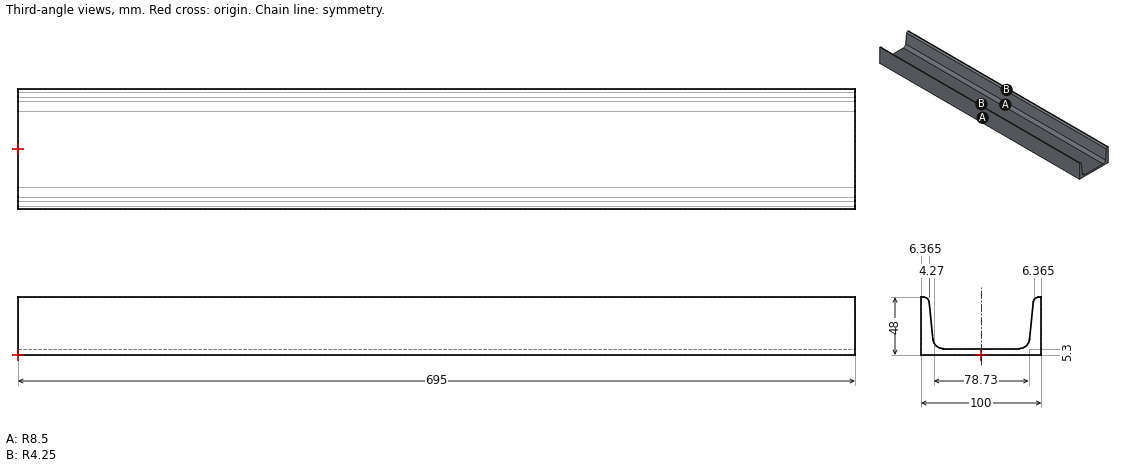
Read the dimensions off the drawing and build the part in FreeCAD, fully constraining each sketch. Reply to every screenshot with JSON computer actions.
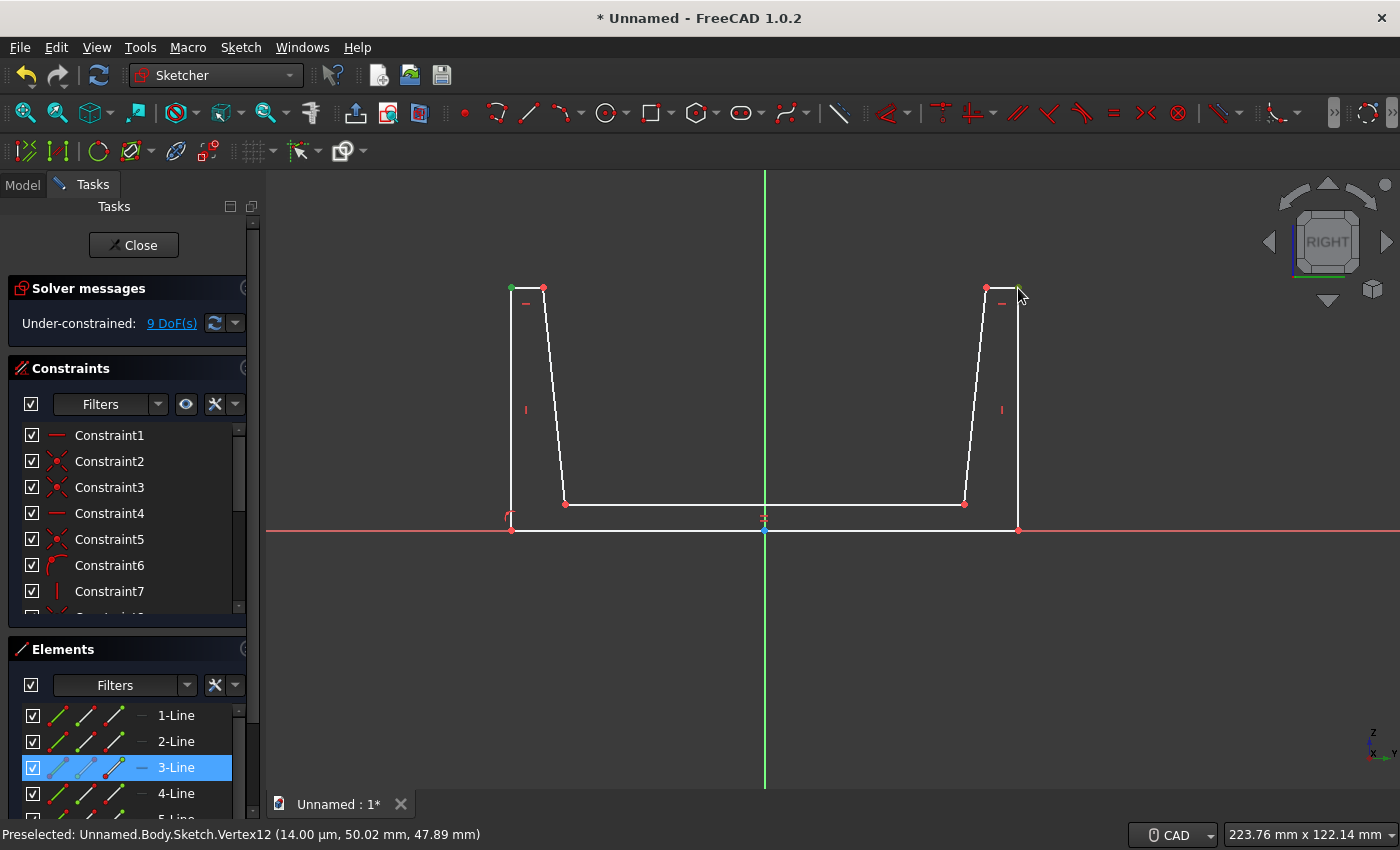
{"action": "left_click", "coordinate": [765, 721]}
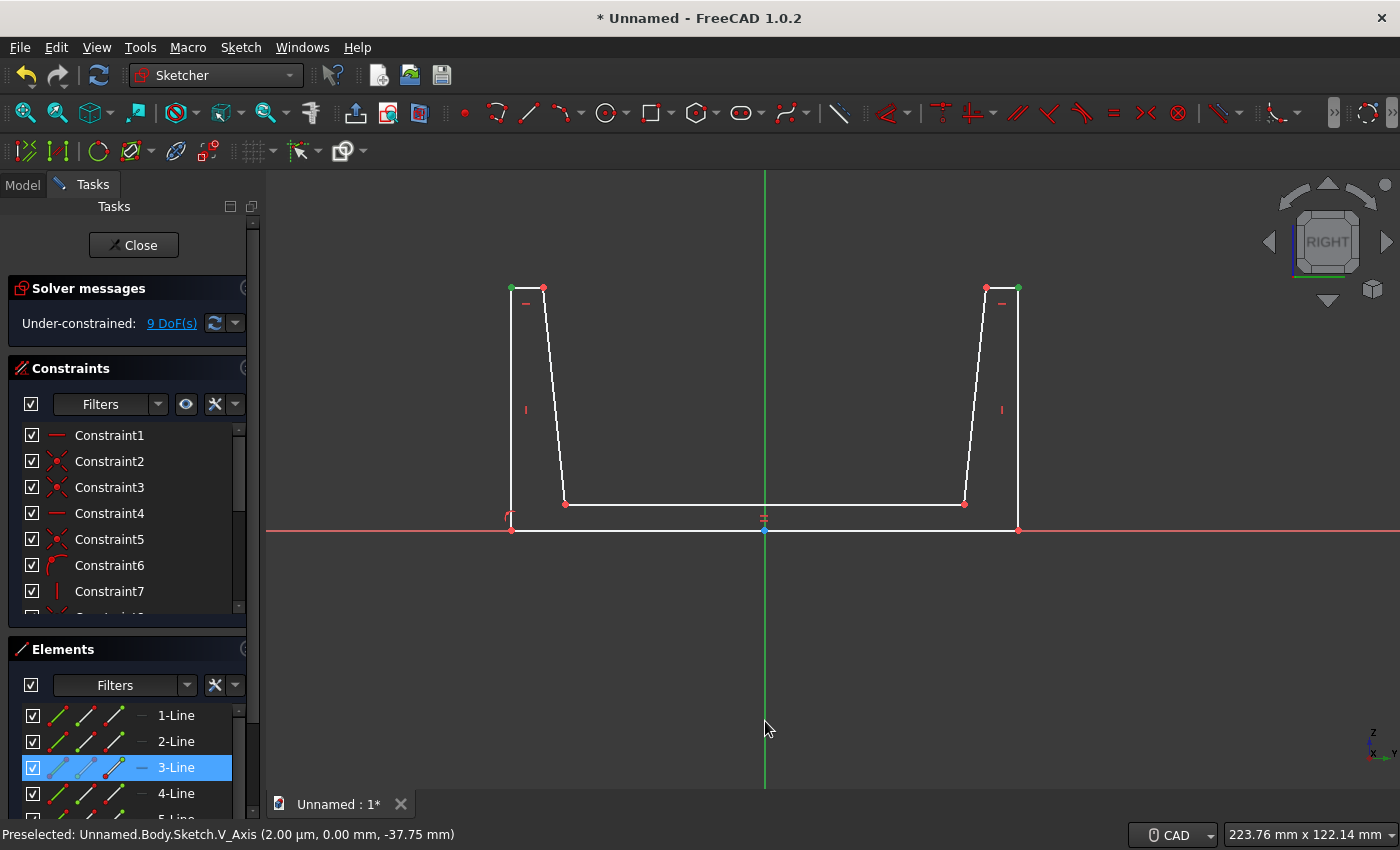
{"action": "key", "text": "s"}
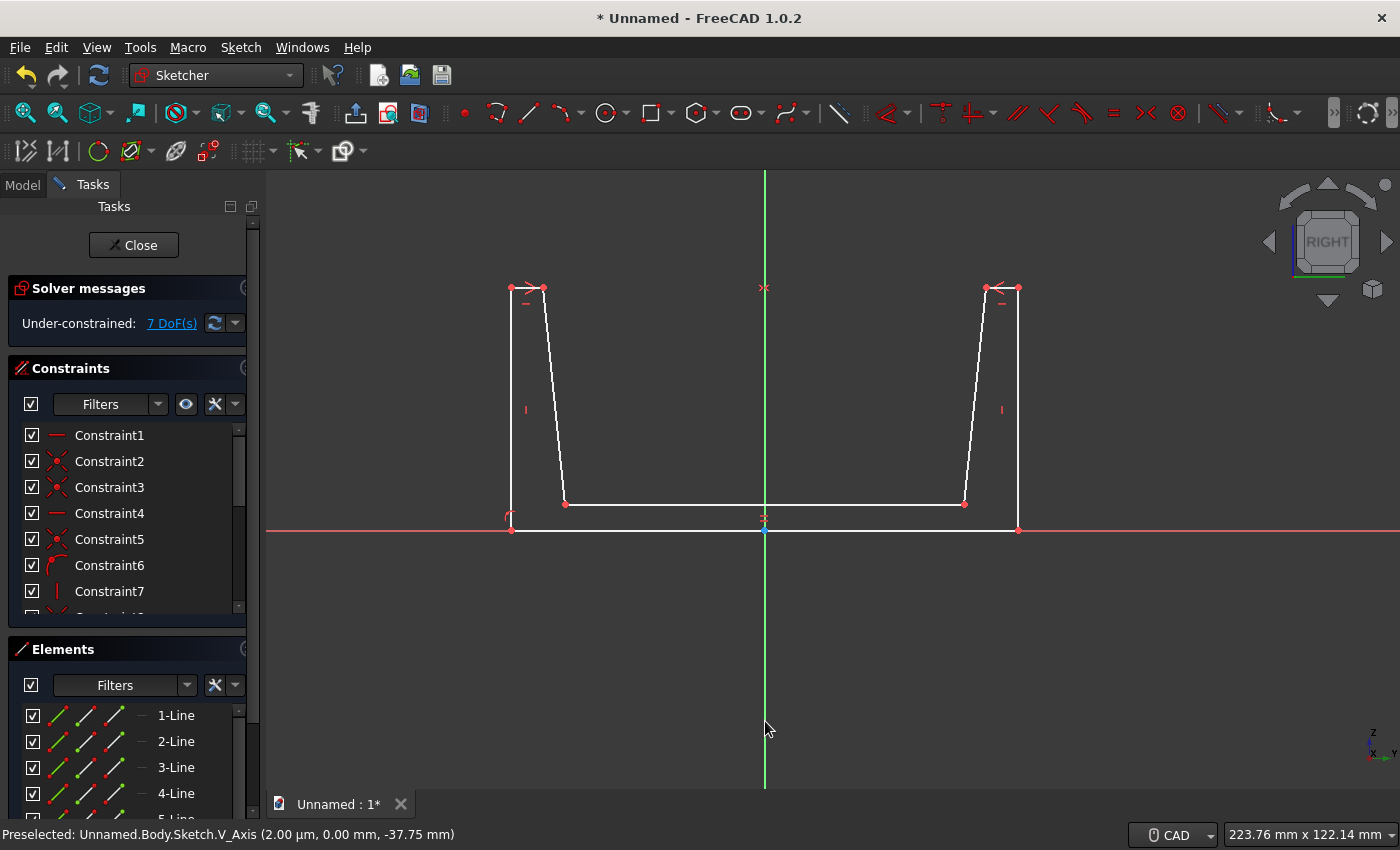
{"action": "left_click", "coordinate": [886, 114]}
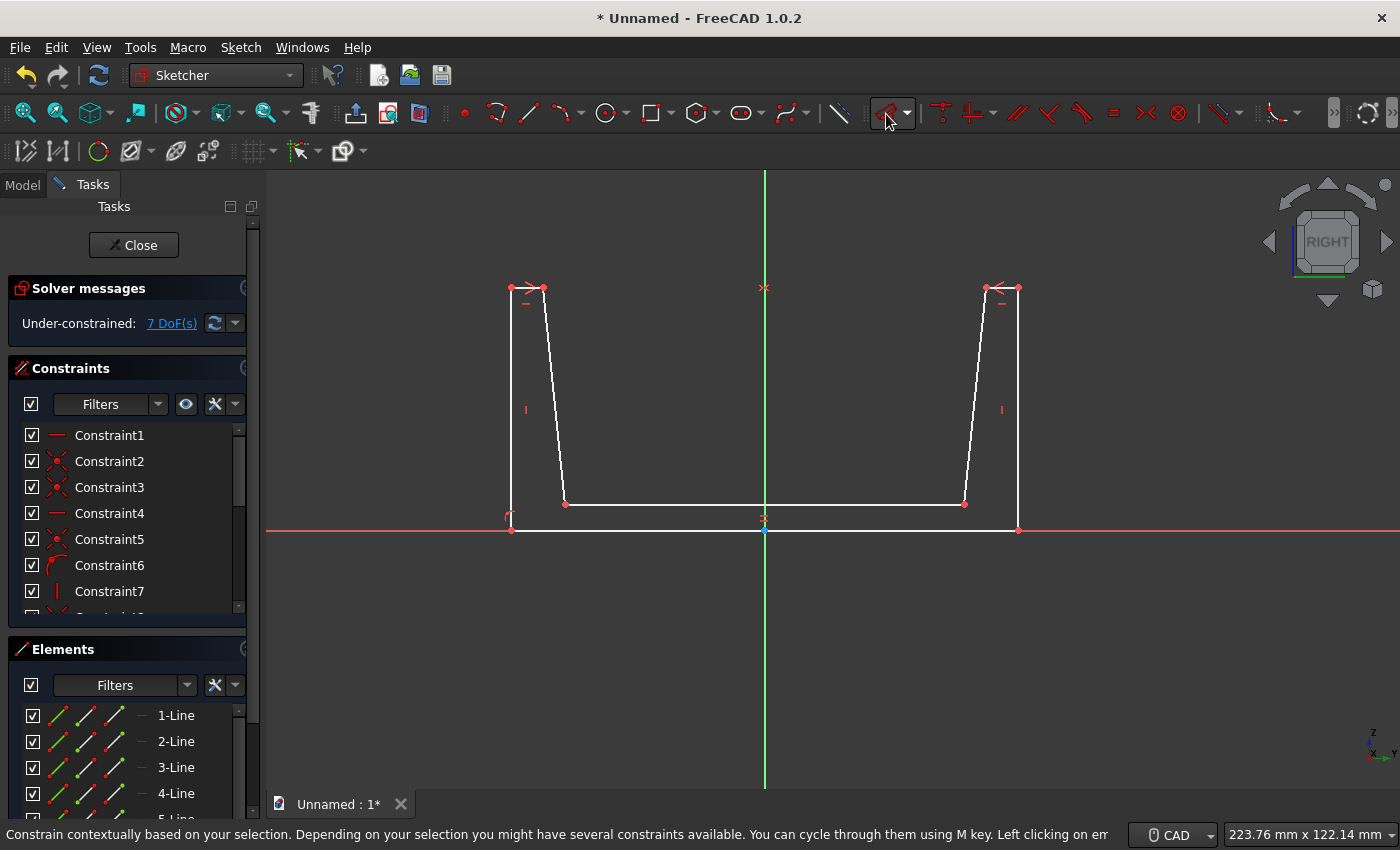
{"action": "left_click", "coordinate": [511, 361]}
{"action": "left_click", "coordinate": [477, 409]}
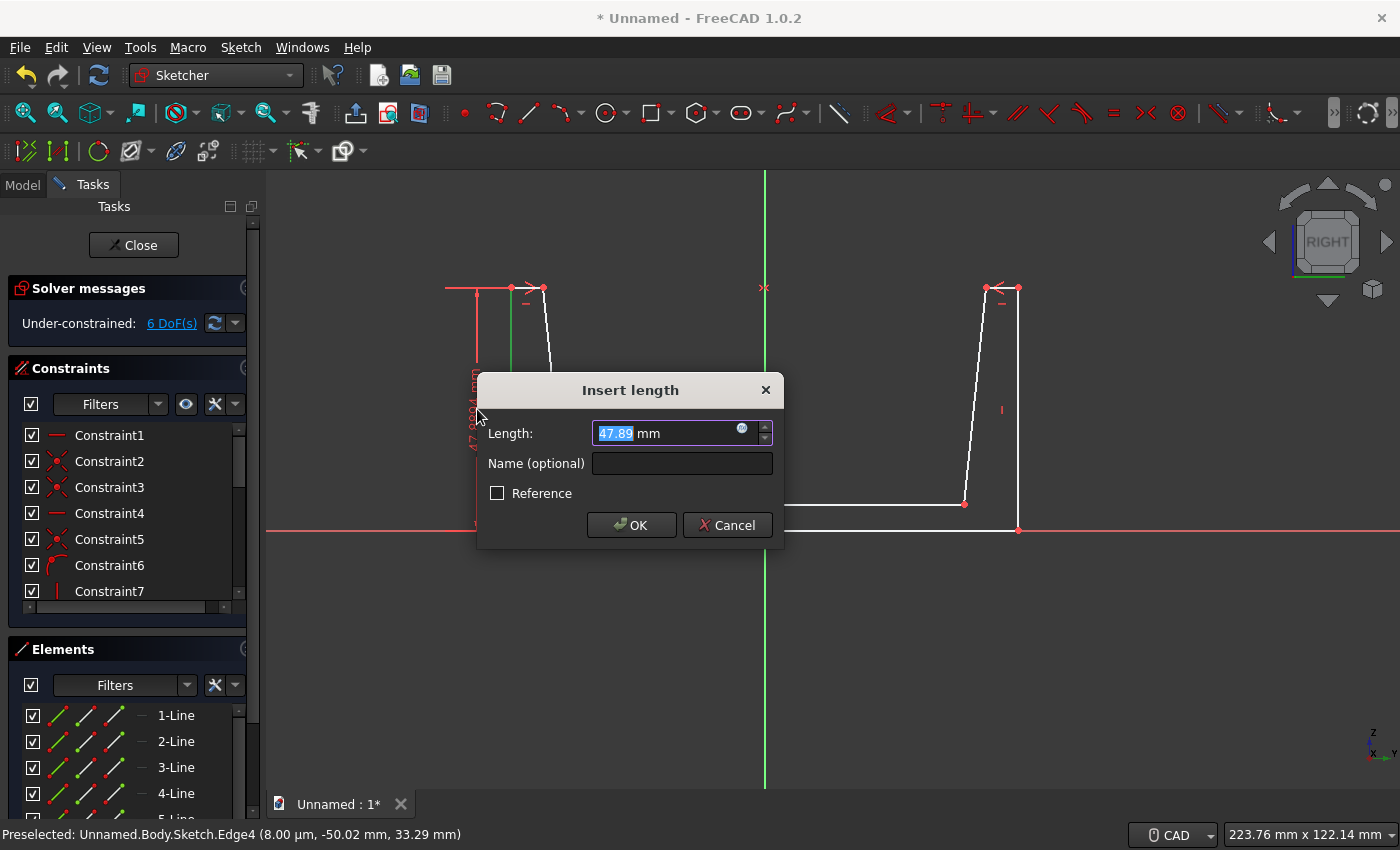
{"action": "type", "text": "48"}
{"action": "key", "text": "Return"}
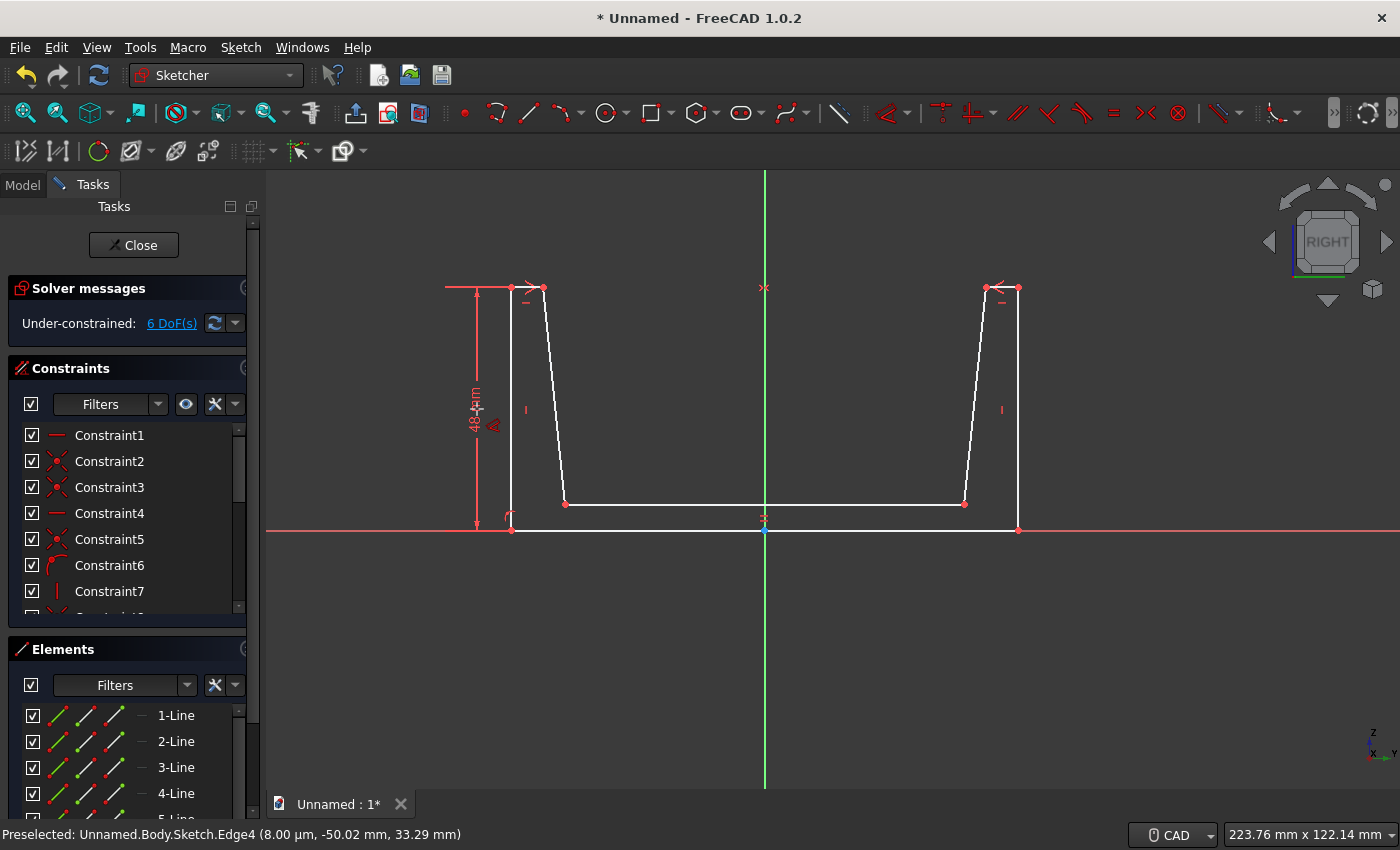
{"action": "left_click", "coordinate": [663, 531]}
{"action": "left_click", "coordinate": [648, 565]}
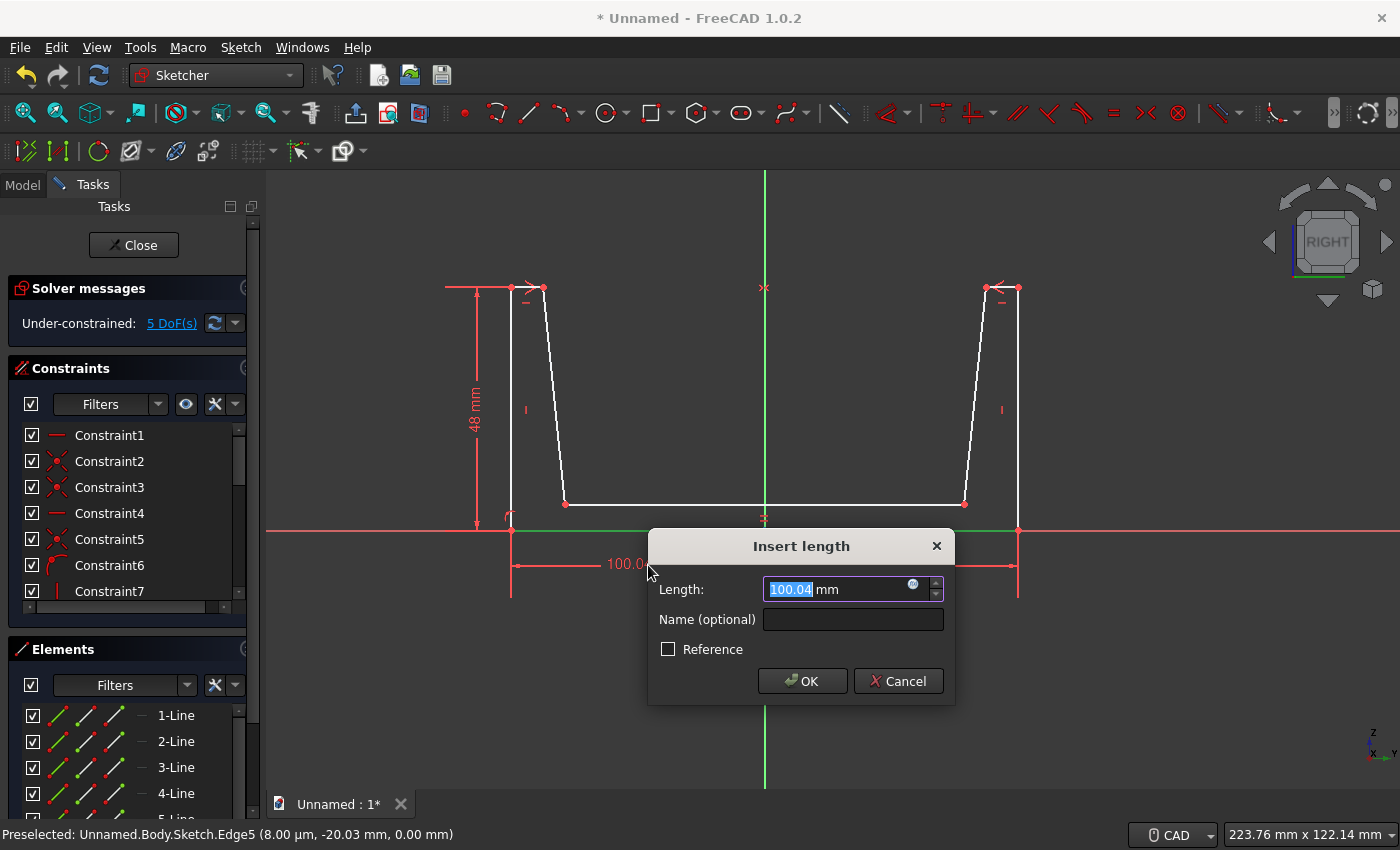
{"action": "type", "text": "100"}
{"action": "key", "text": "Return"}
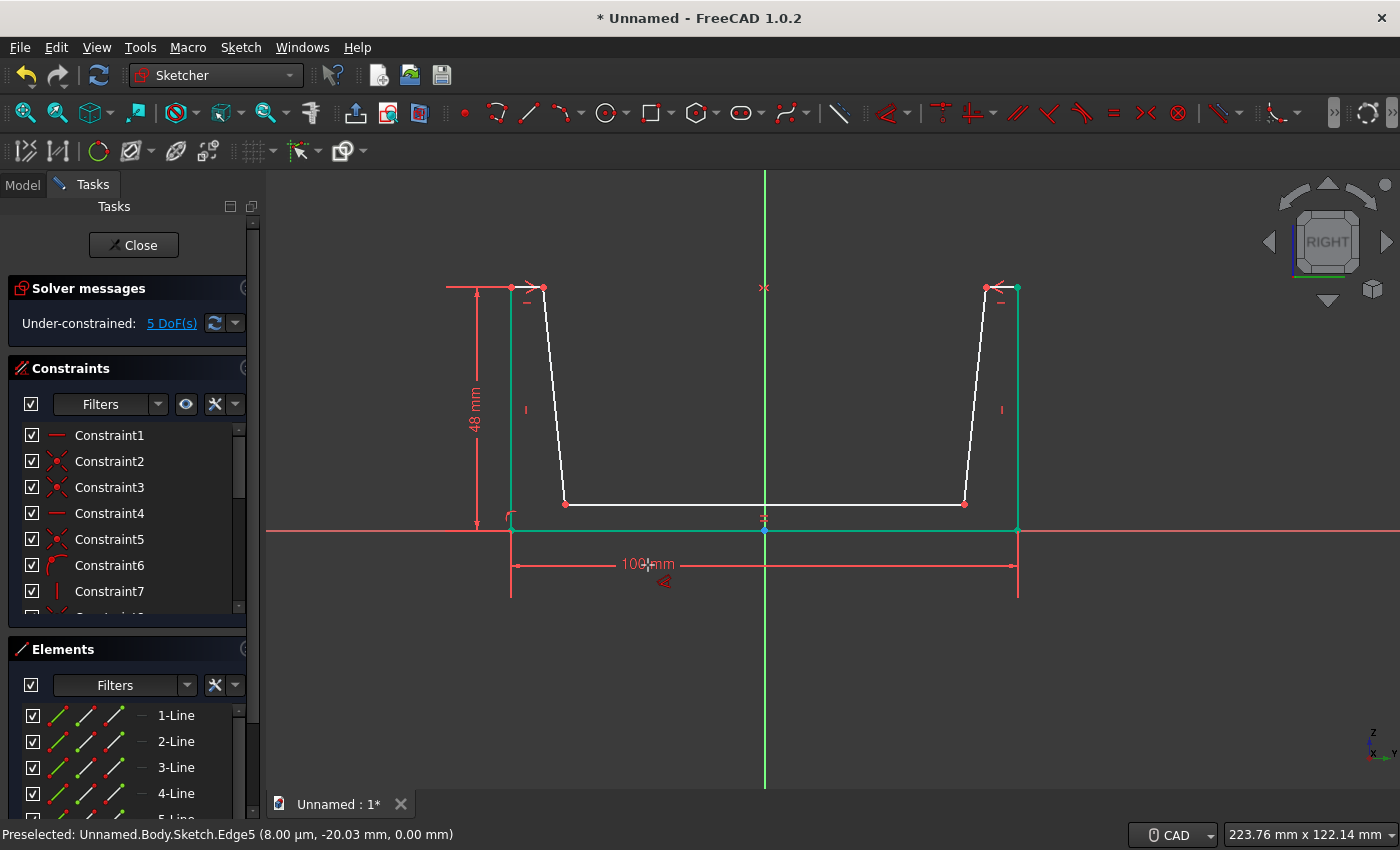
{"action": "scroll", "coordinate": [964, 505], "scroll_direction": "up", "scroll_amount": 2}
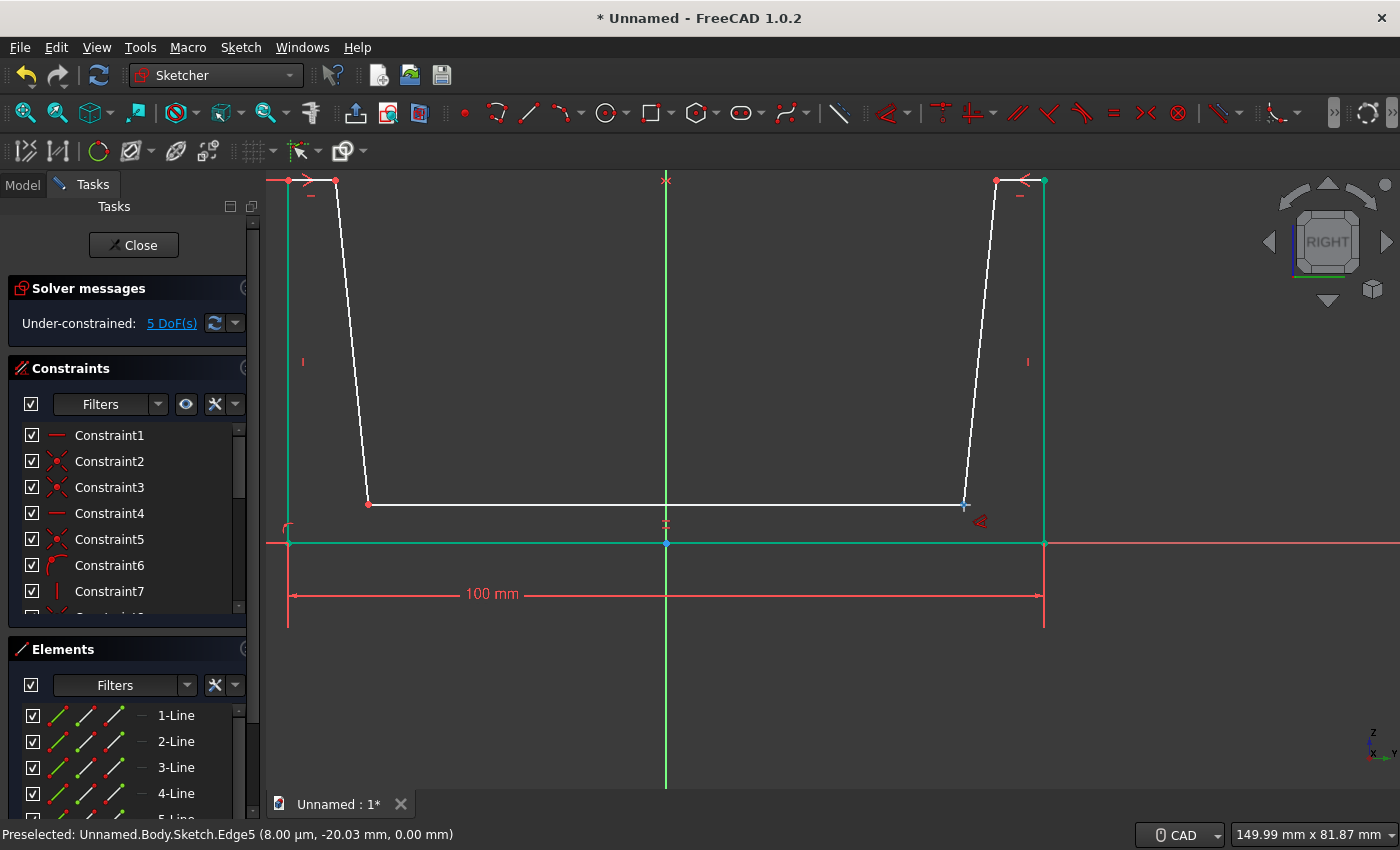
{"action": "left_click", "coordinate": [964, 505]}
{"action": "left_click", "coordinate": [998, 524]}